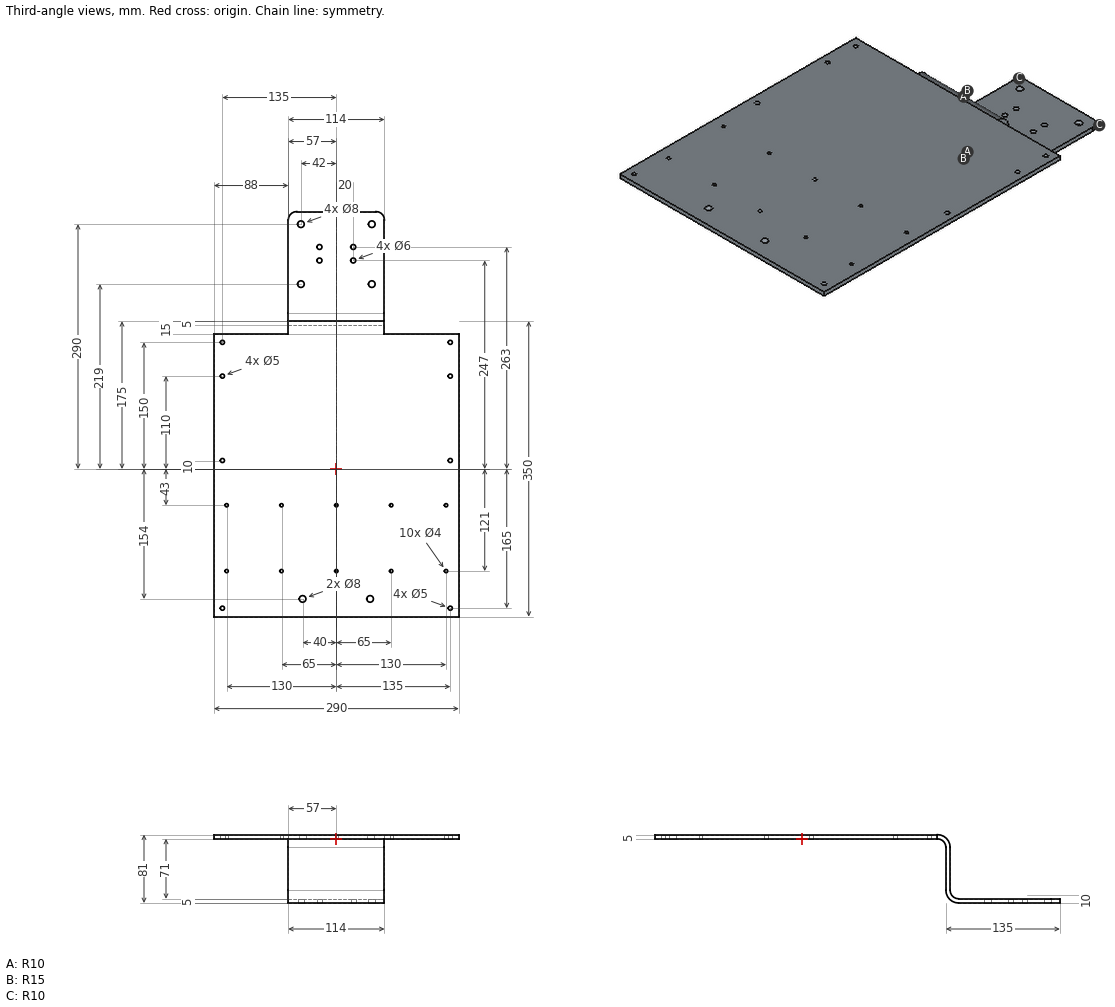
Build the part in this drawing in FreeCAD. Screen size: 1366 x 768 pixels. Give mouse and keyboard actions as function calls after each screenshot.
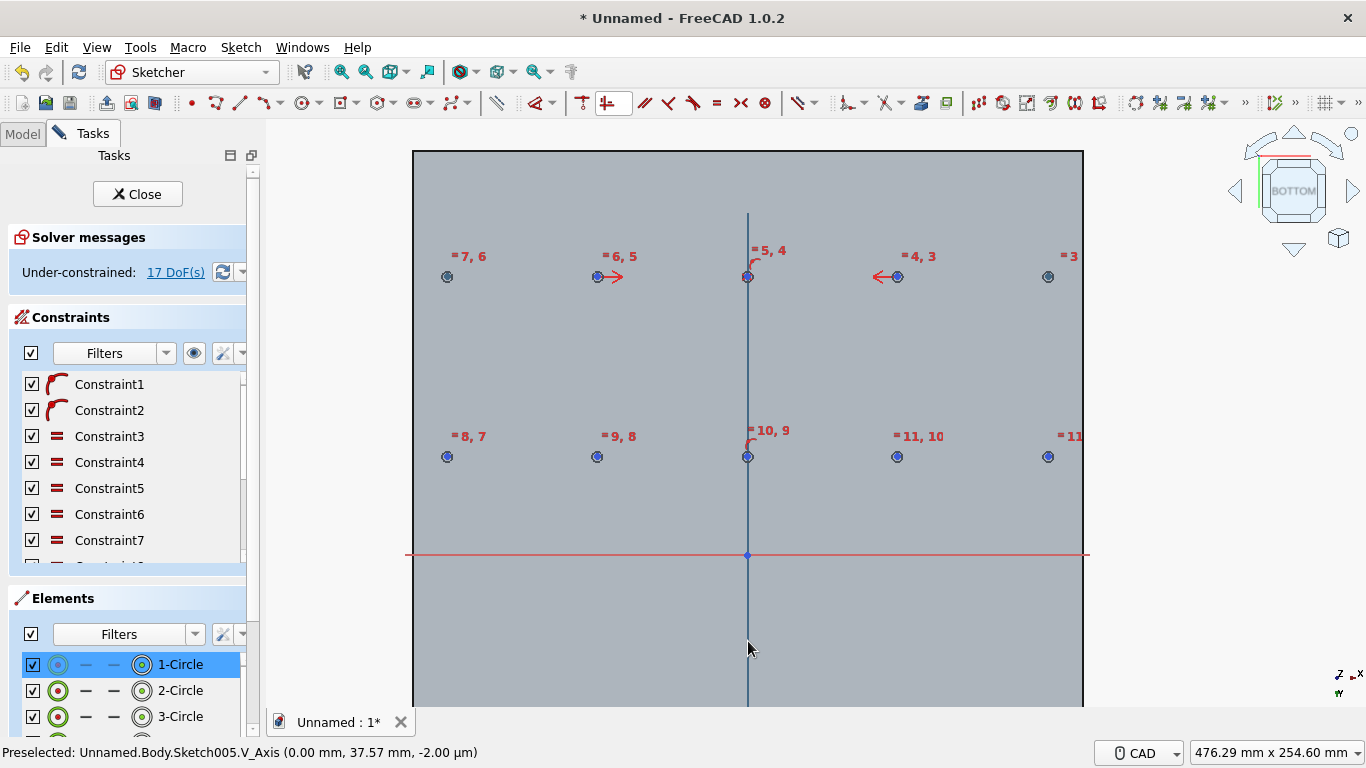
click(742, 104)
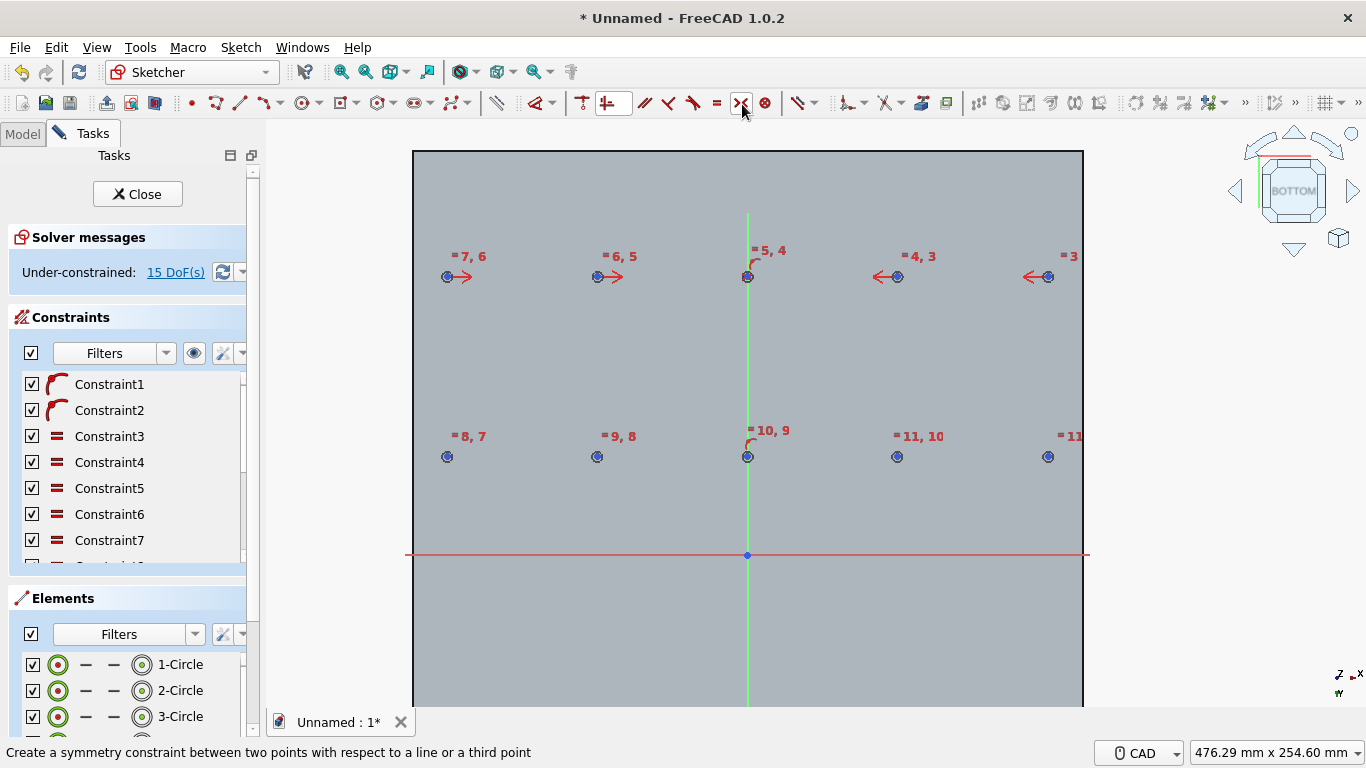
click(597, 457)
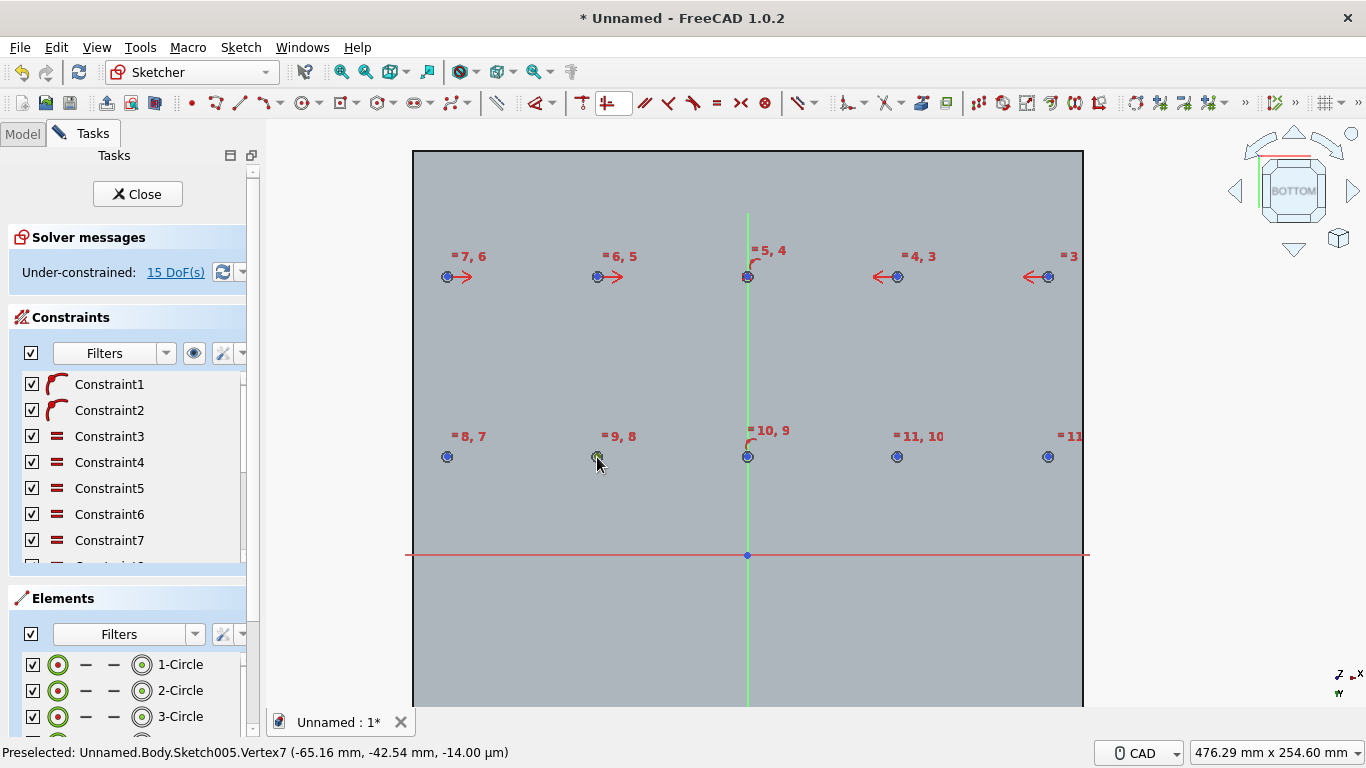
click(897, 457)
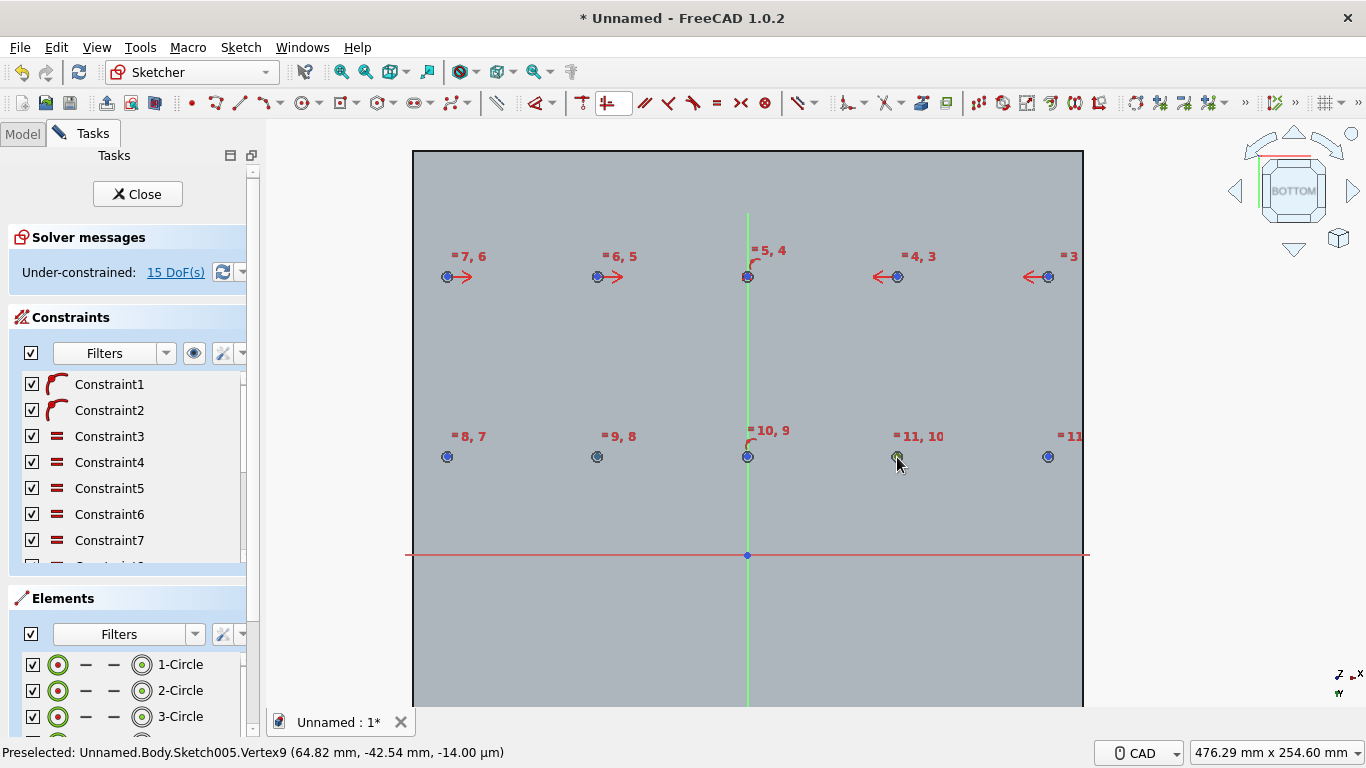
click(748, 641)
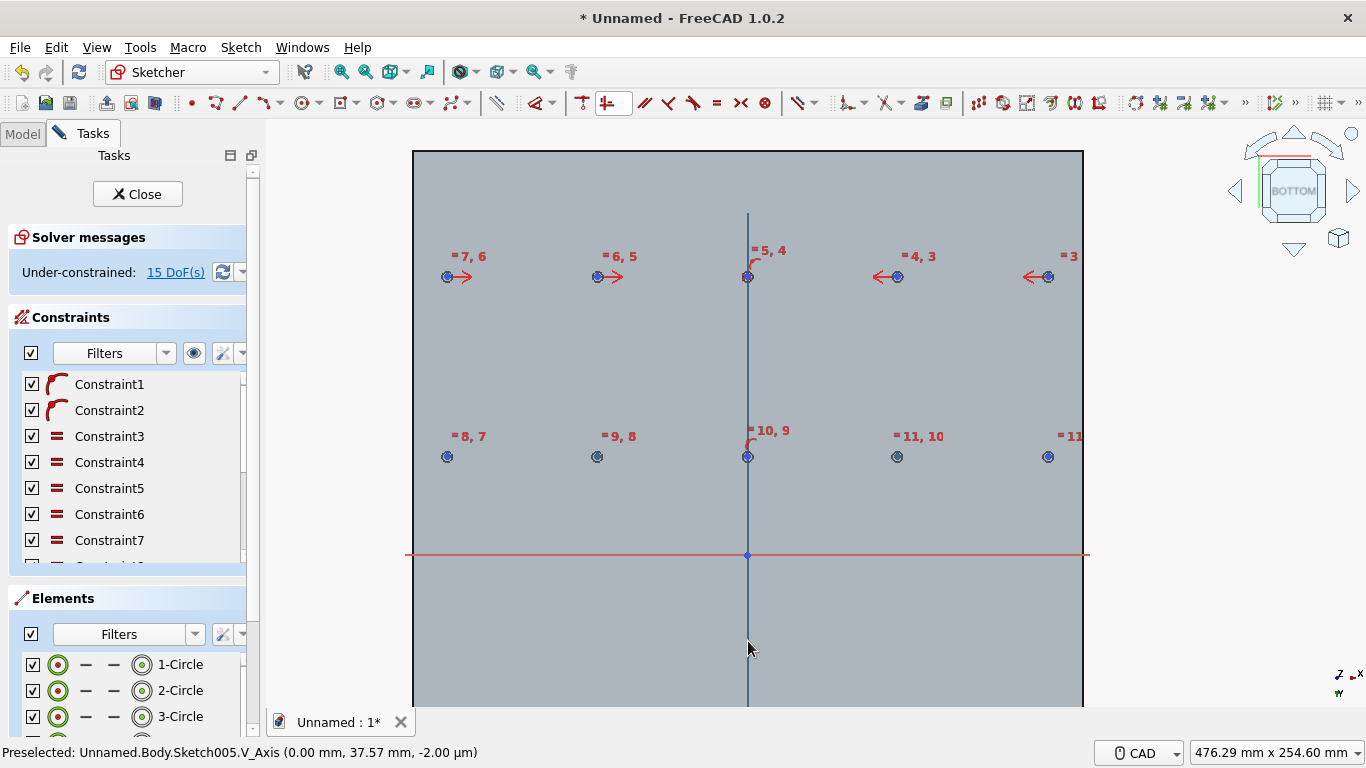
key(s)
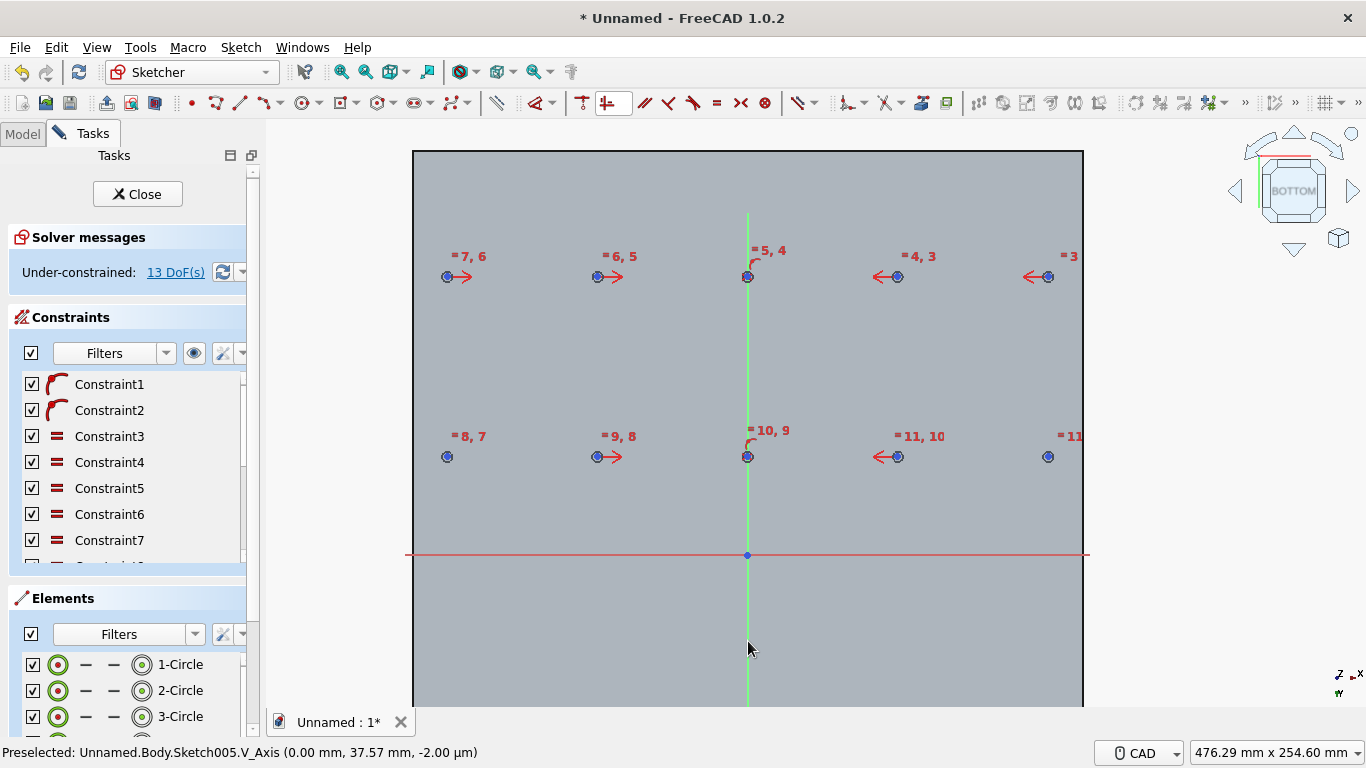
click(447, 457)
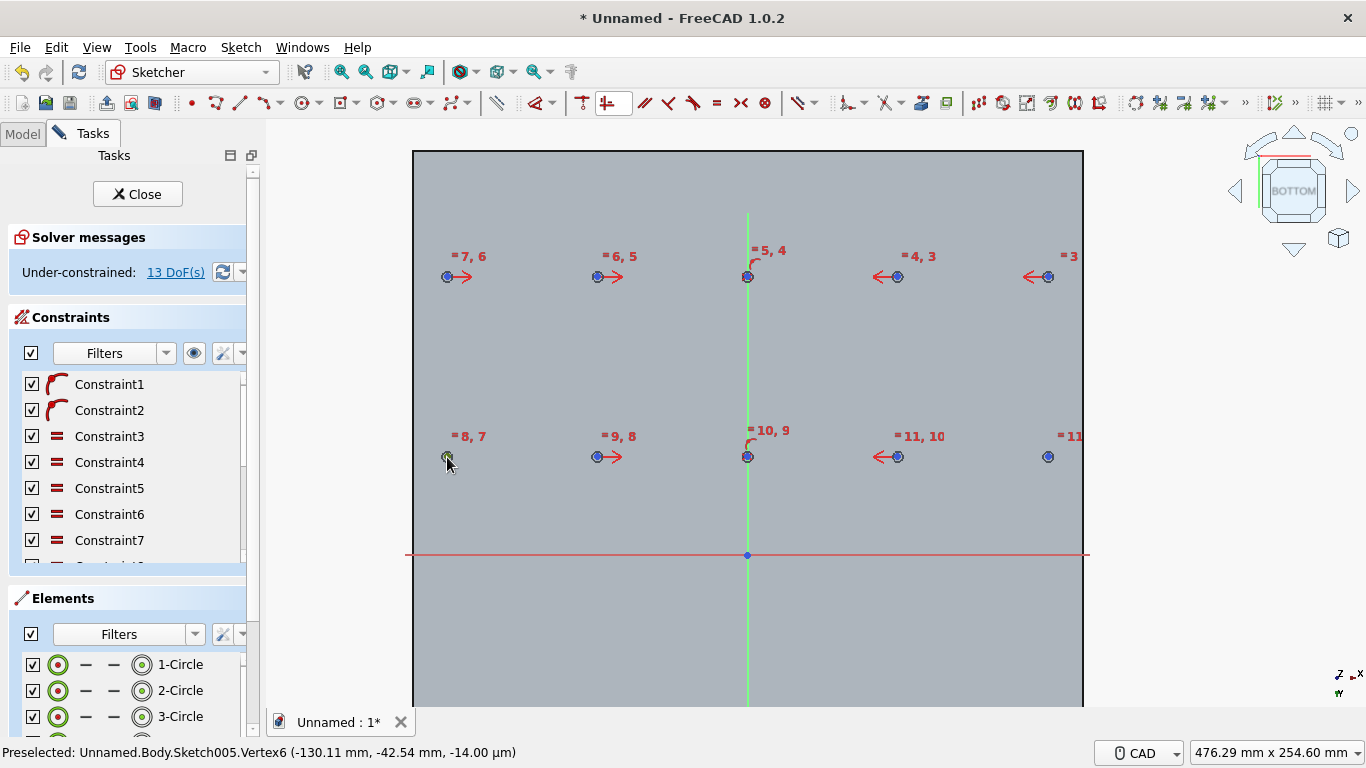
click(1048, 457)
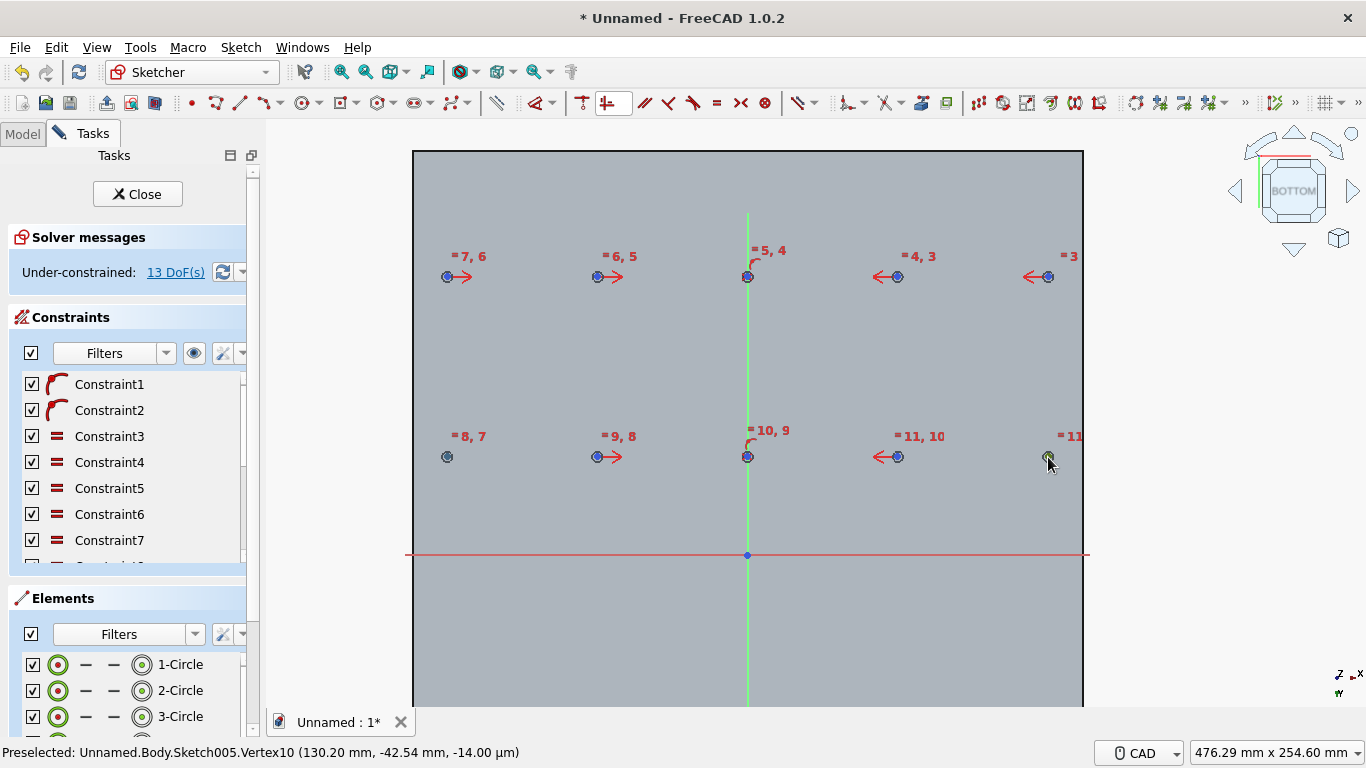
click(748, 641)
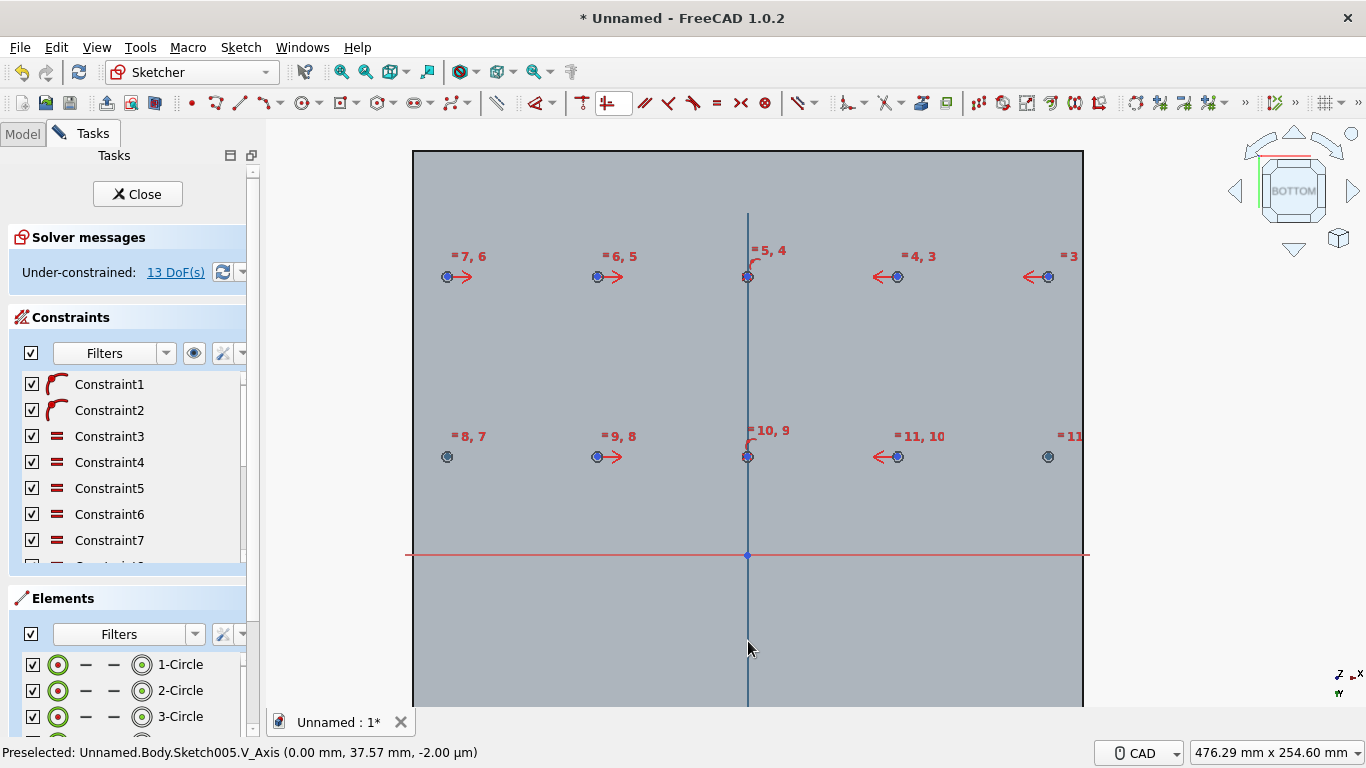
click(742, 104)